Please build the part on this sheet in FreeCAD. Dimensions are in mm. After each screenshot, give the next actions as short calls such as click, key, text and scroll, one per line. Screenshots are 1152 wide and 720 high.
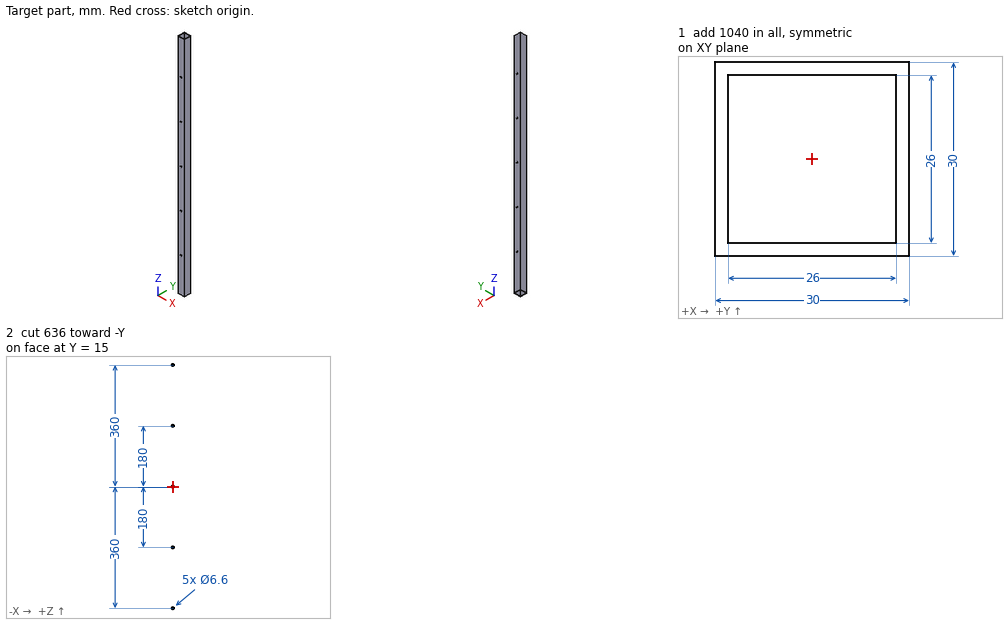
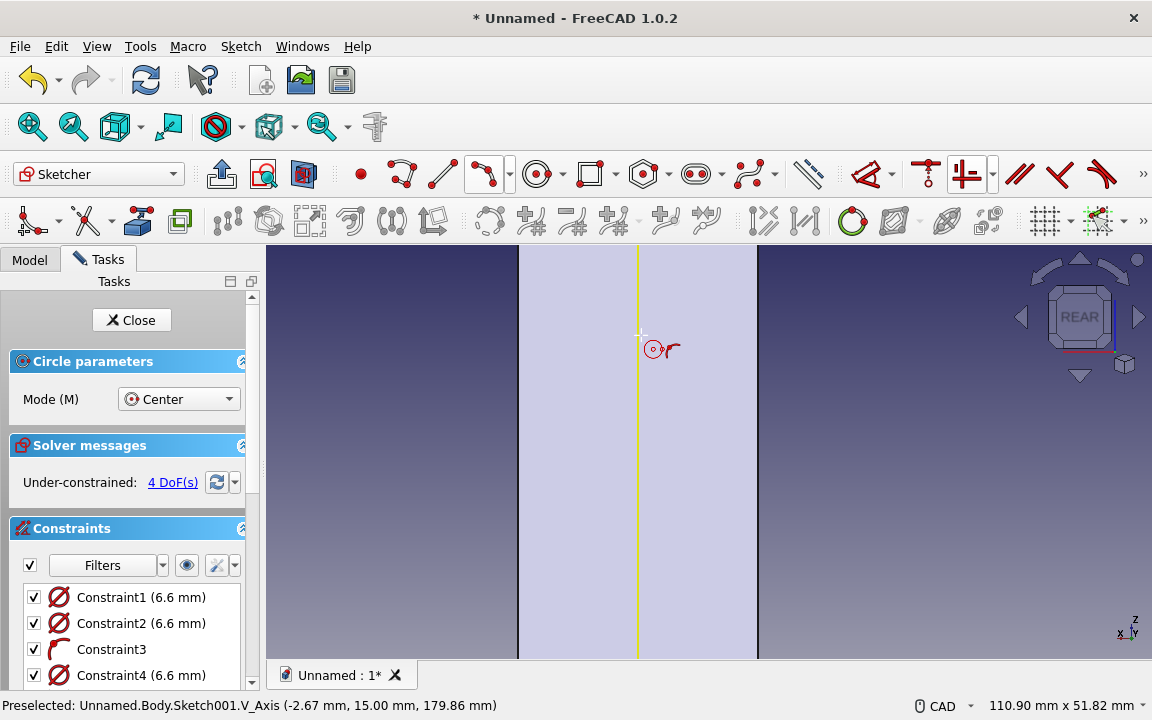
scroll(641, 308, down, 15)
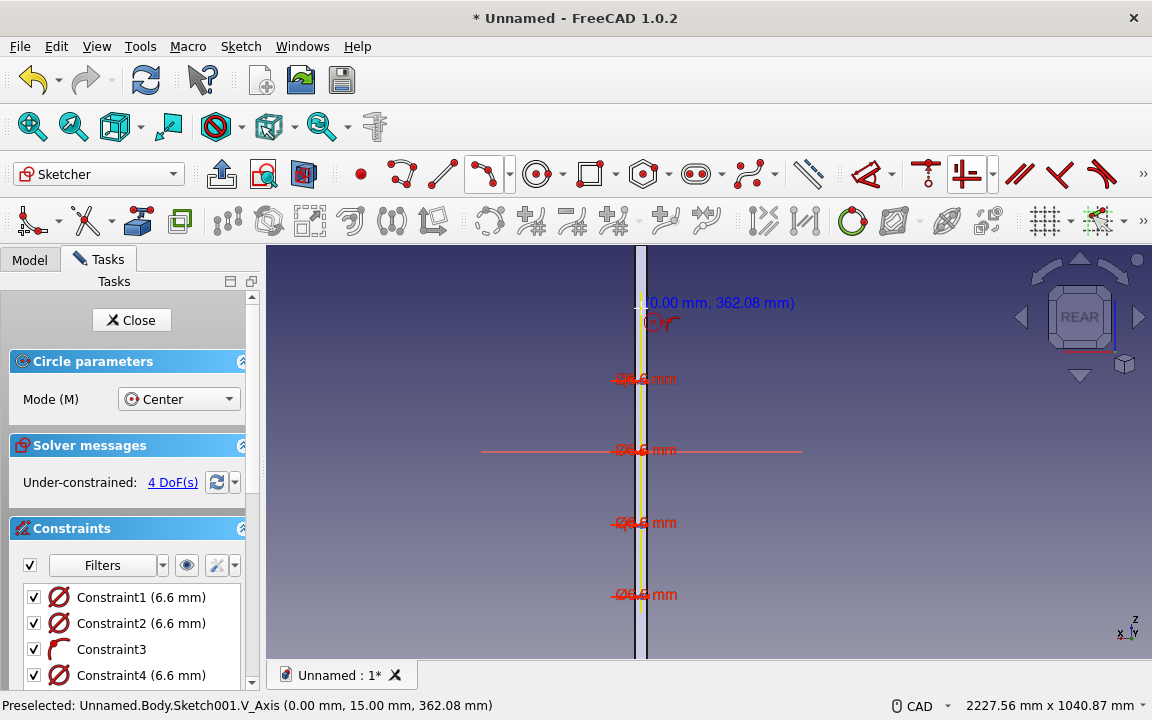
click(641, 309)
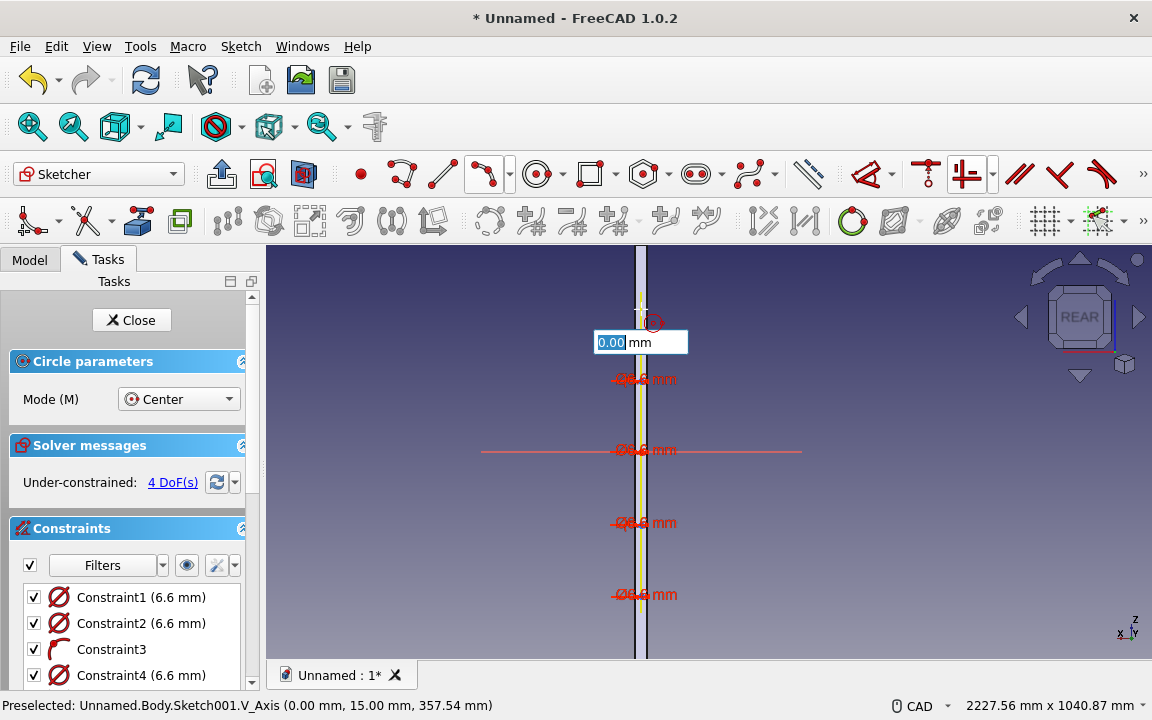
scroll(642, 309, up, 13)
move(643, 301)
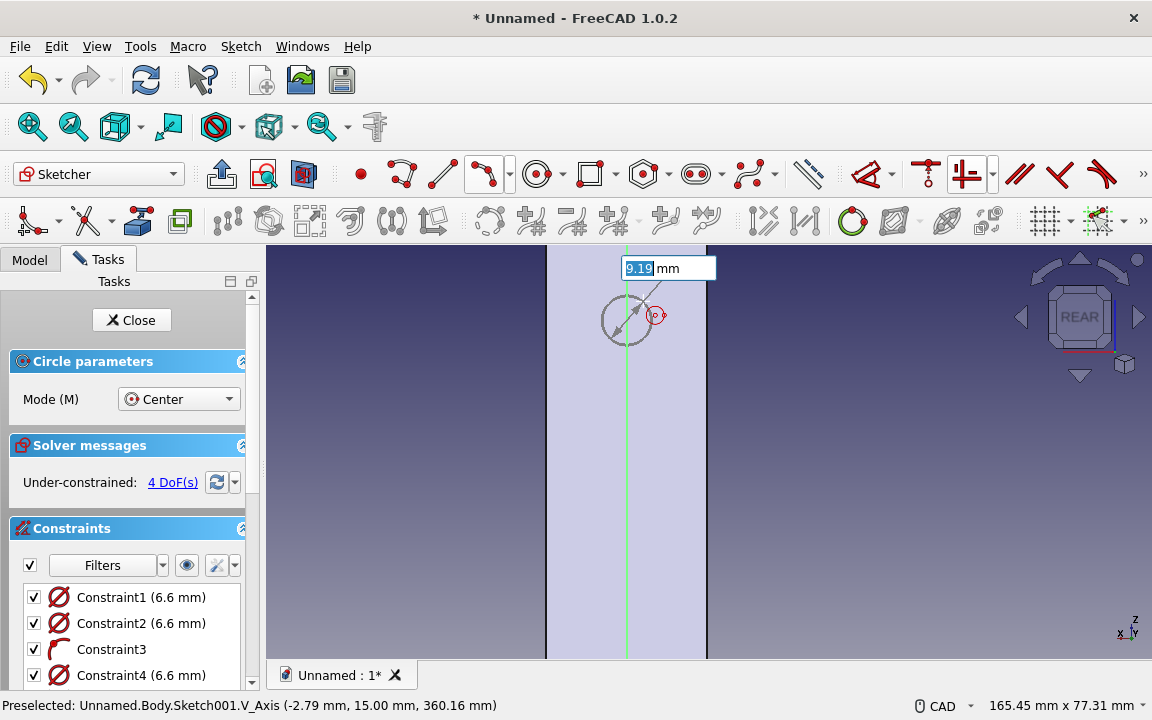
text(6.6)
key(Return)
key(Escape)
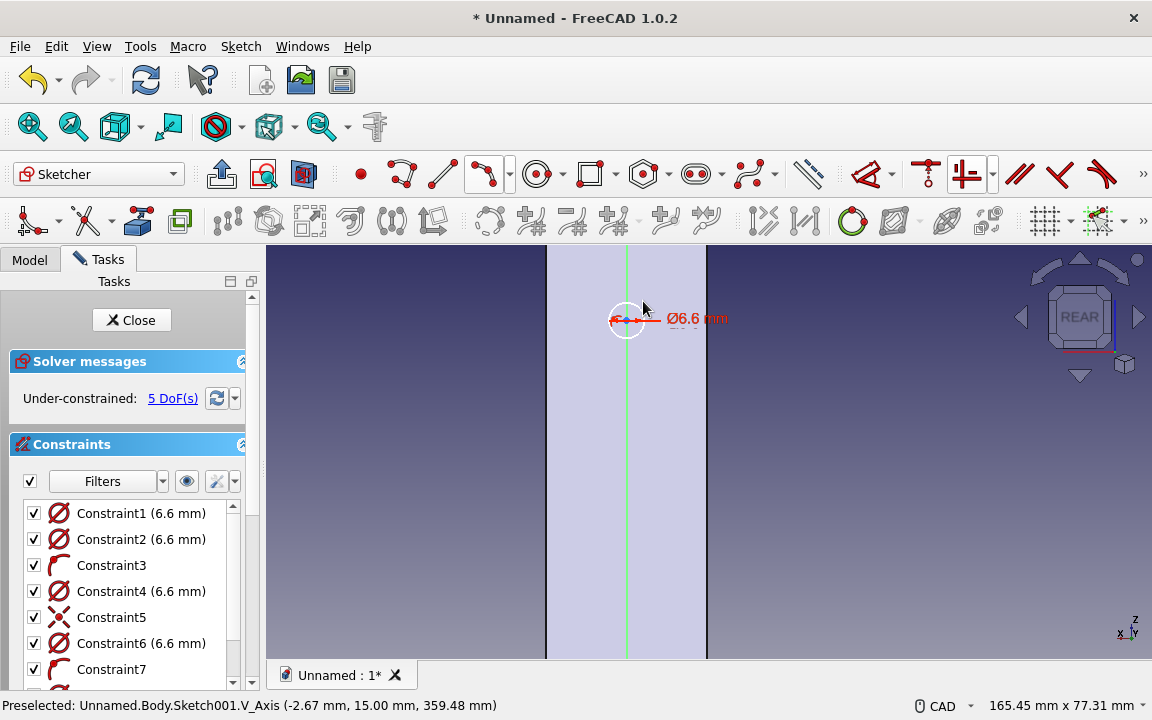
scroll(641, 337, down, 14)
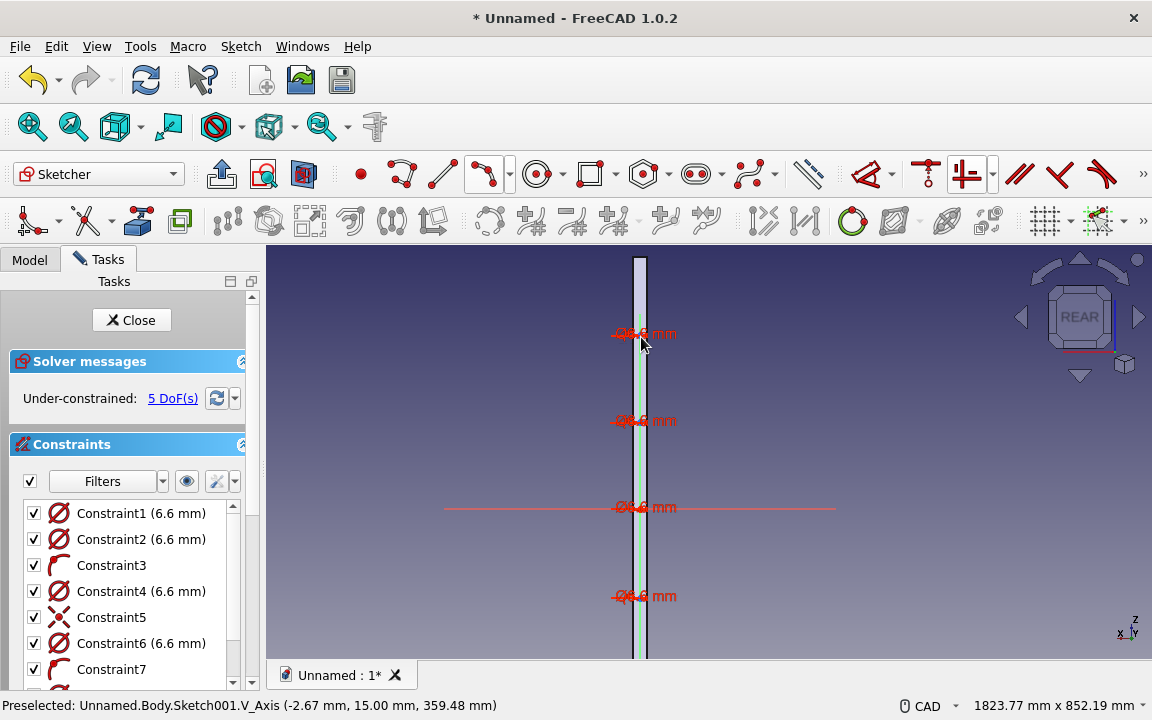
click(641, 571)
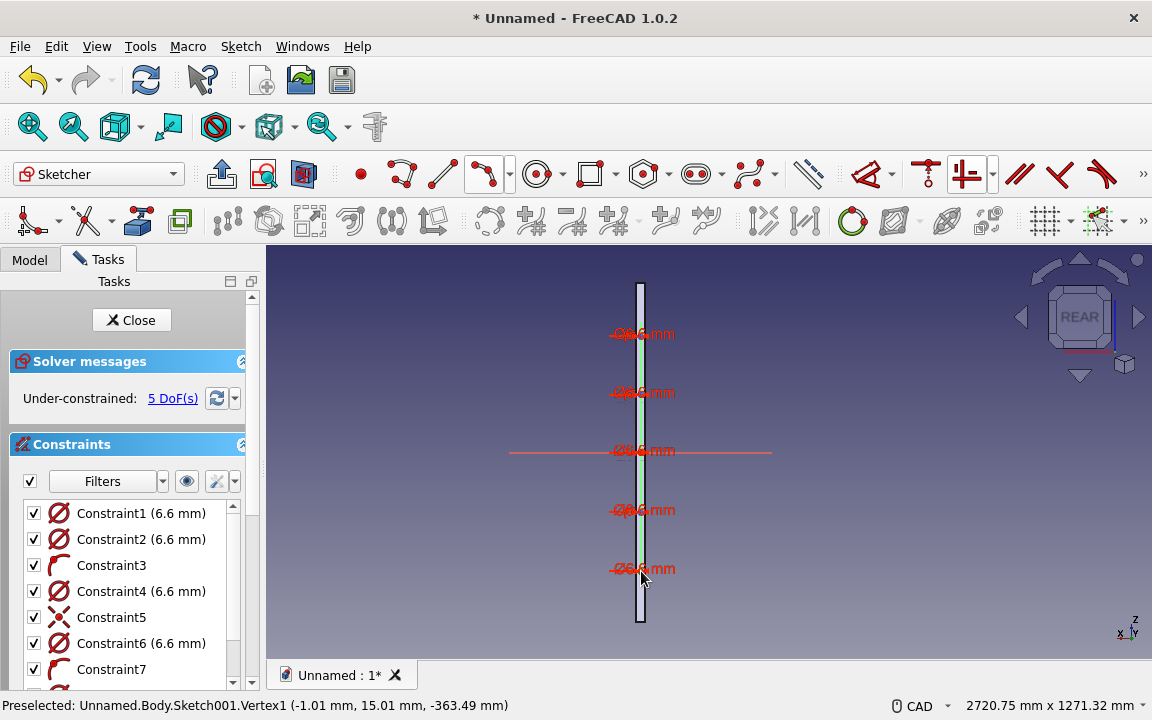
click(641, 426)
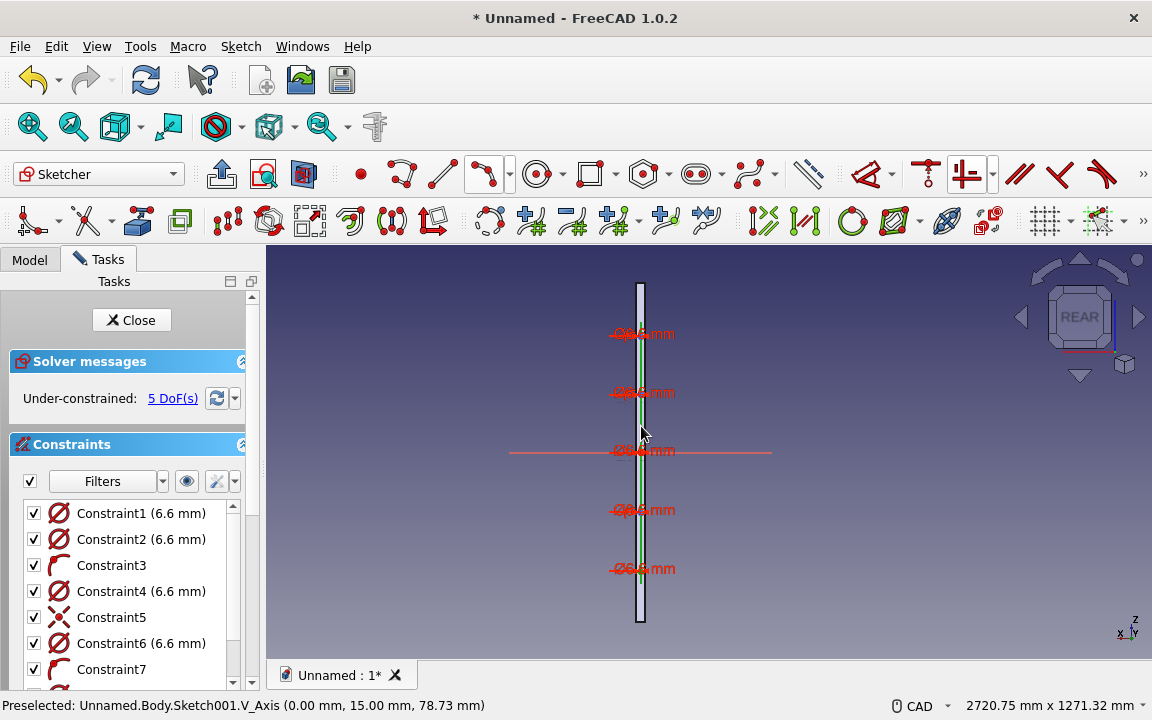
key(c)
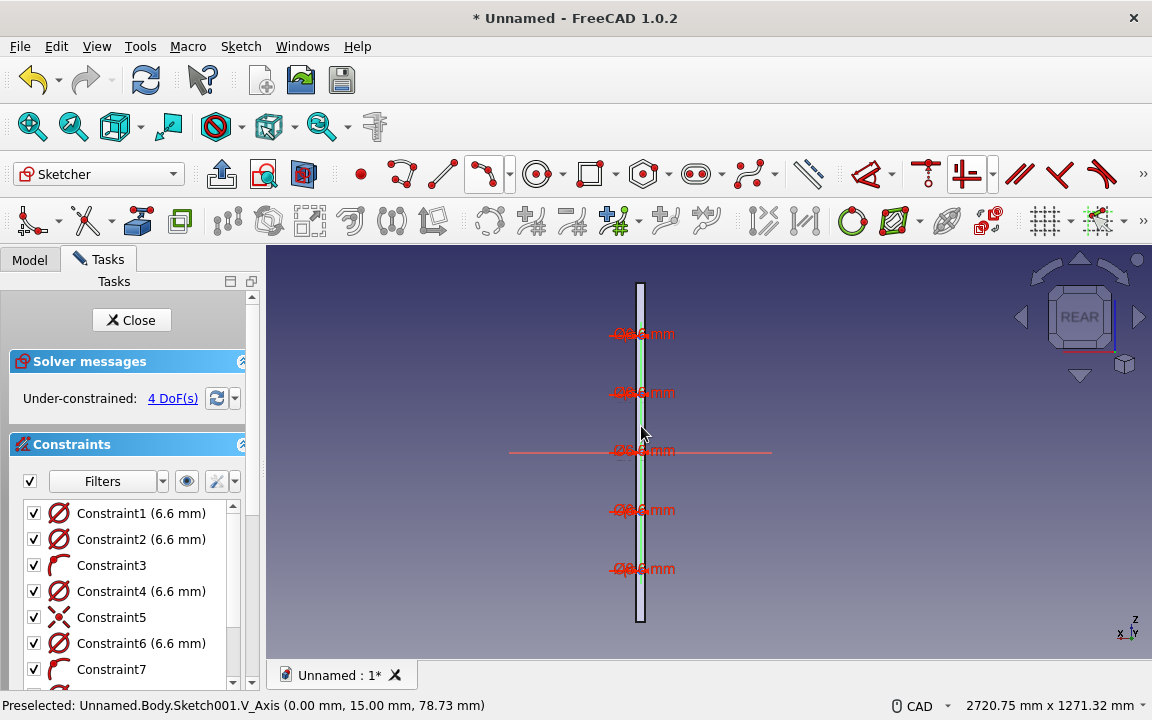
key(d)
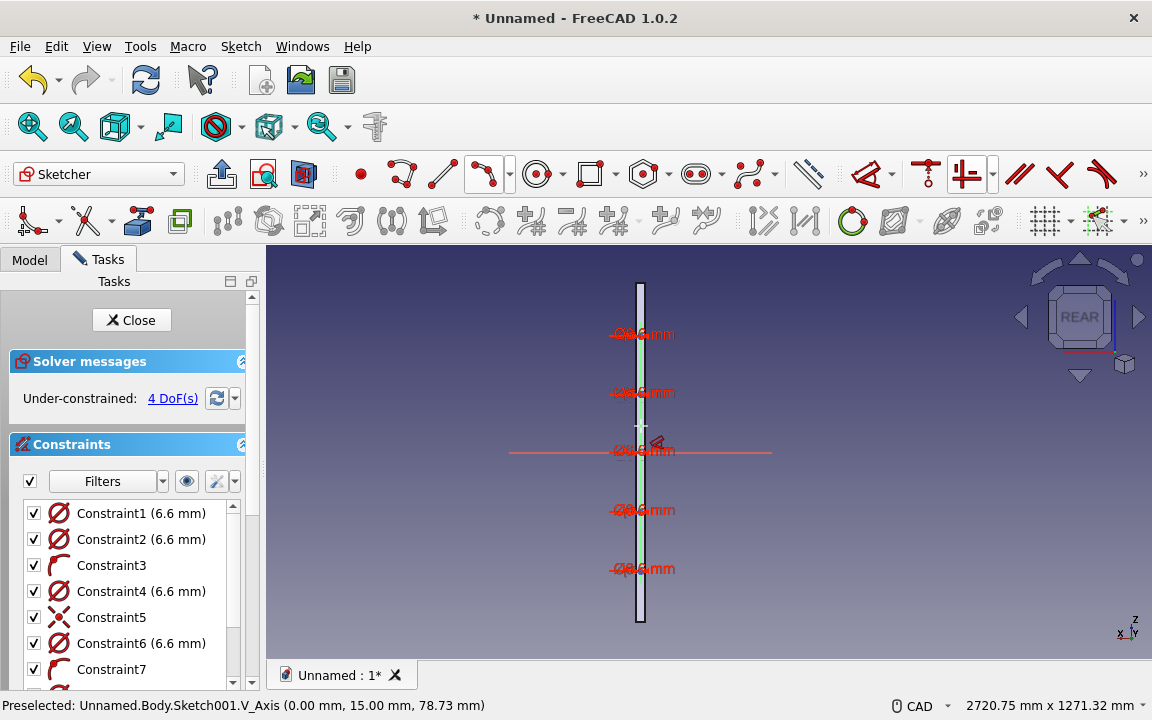
click(641, 571)
click(675, 512)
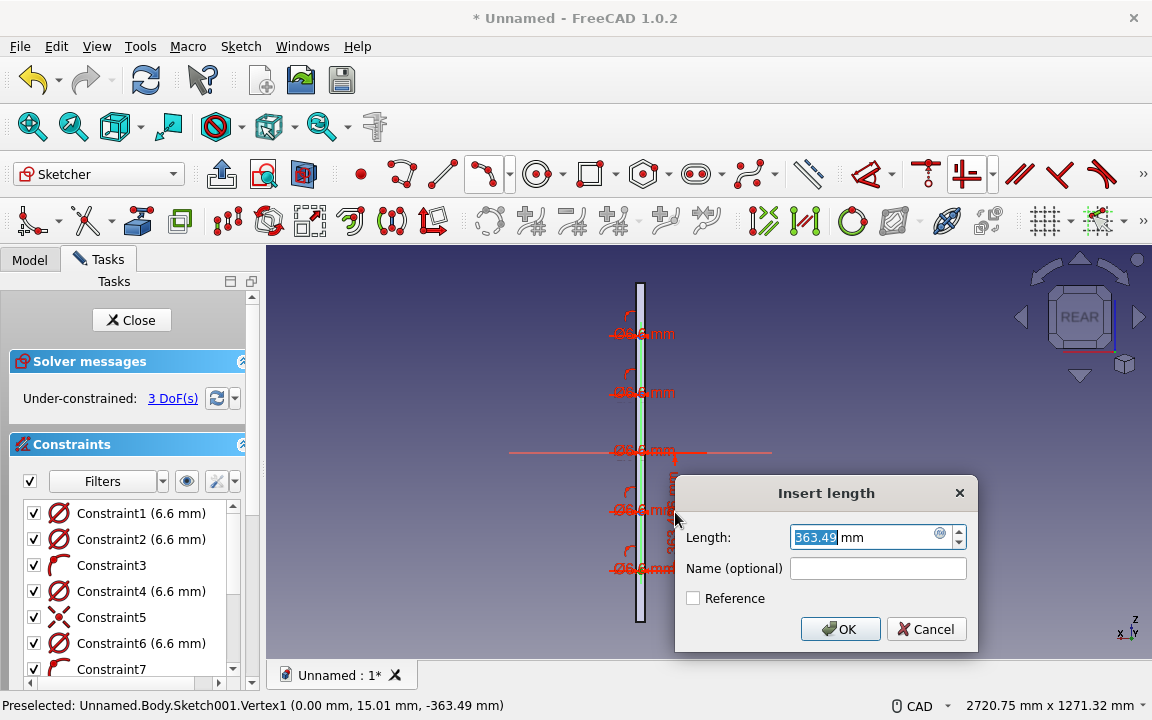
text(360)
key(Return)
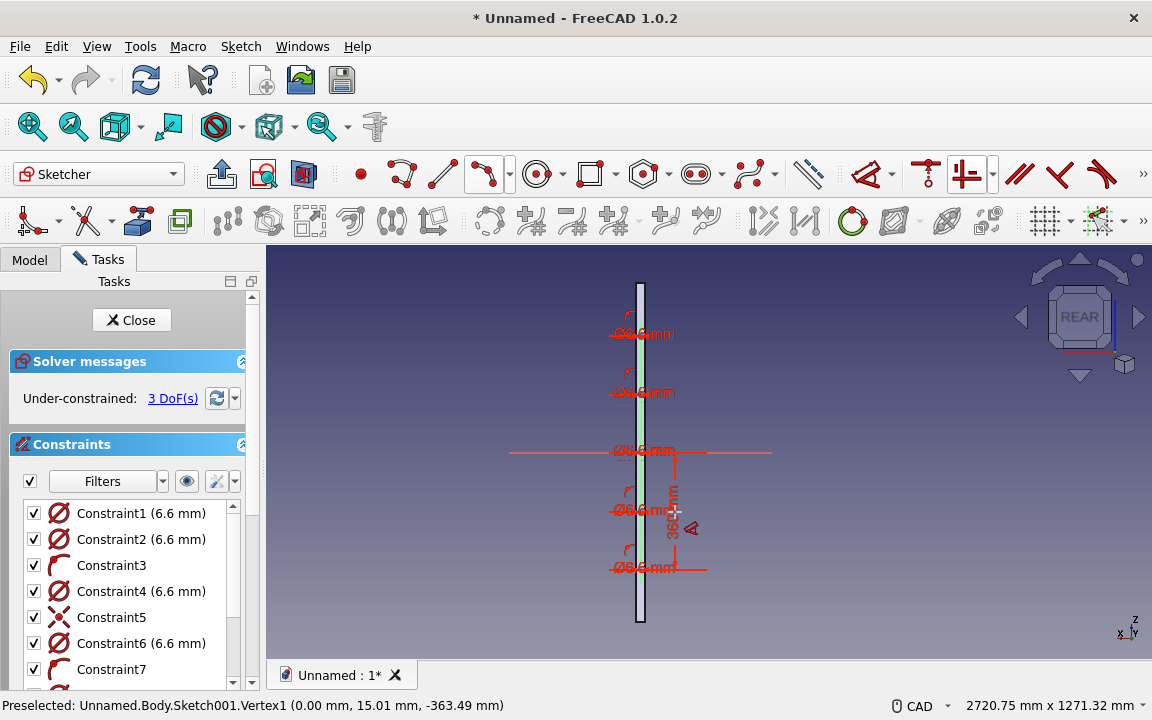
click(641, 512)
click(675, 482)